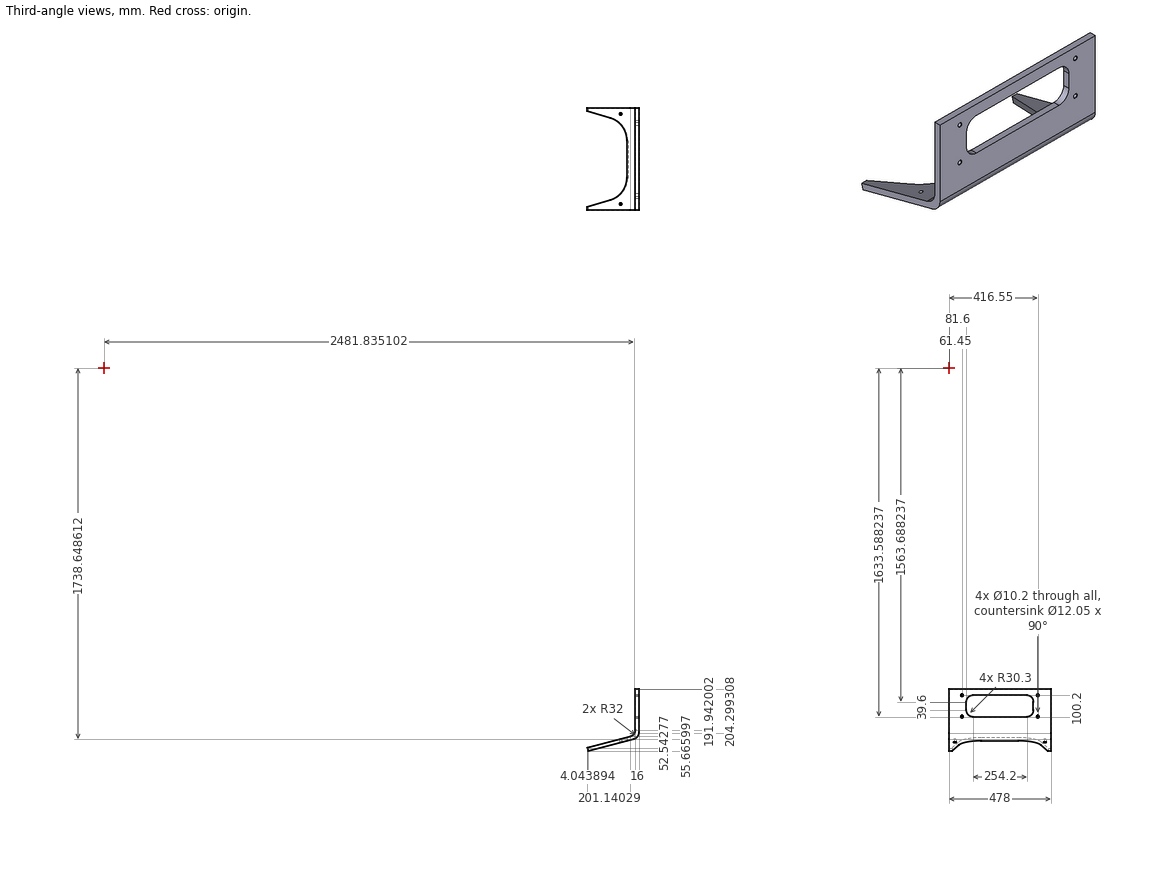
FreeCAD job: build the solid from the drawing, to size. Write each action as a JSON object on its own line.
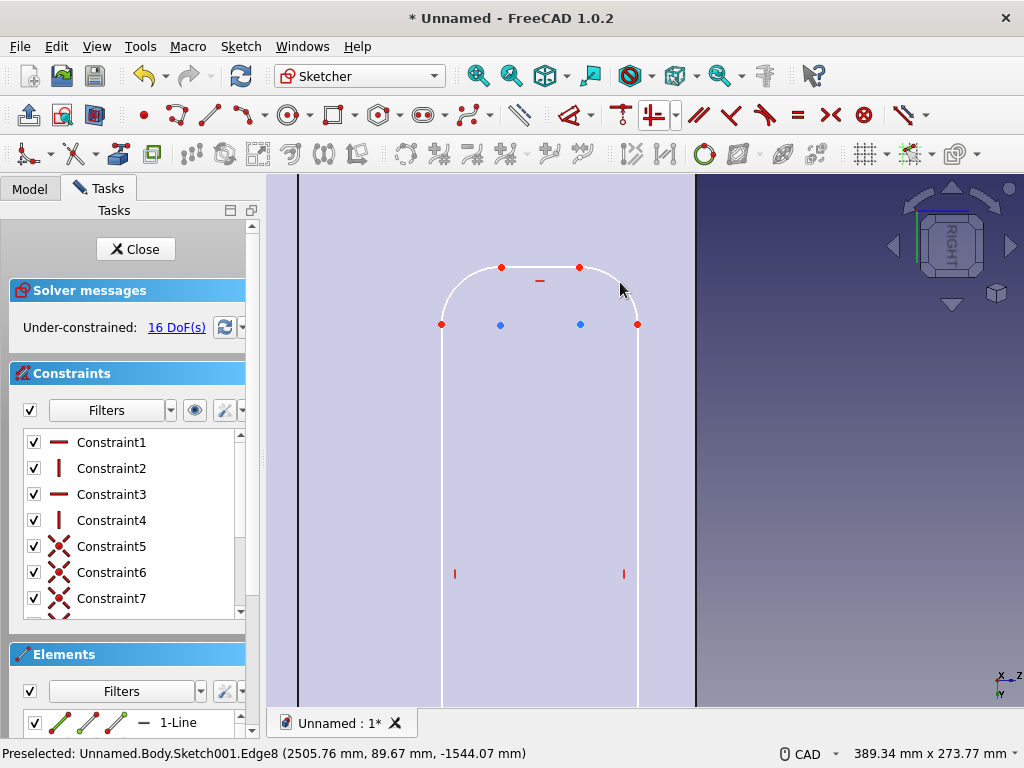
{"action": "left_click", "coordinate": [556, 267]}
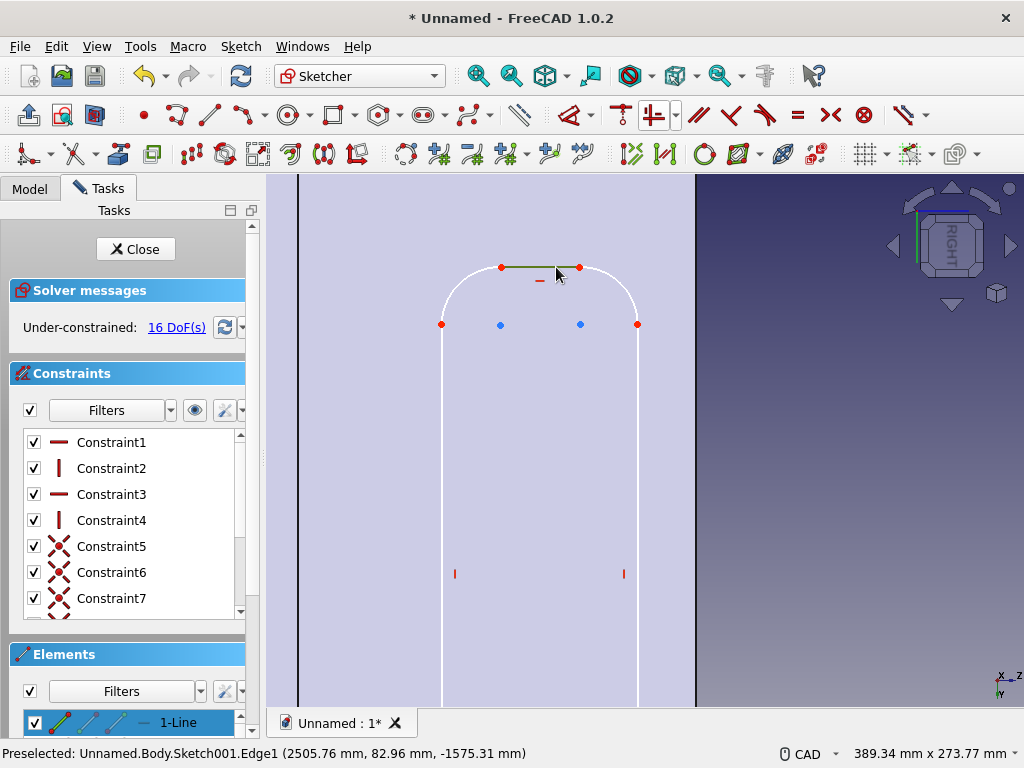
{"action": "left_click", "coordinate": [475, 273]}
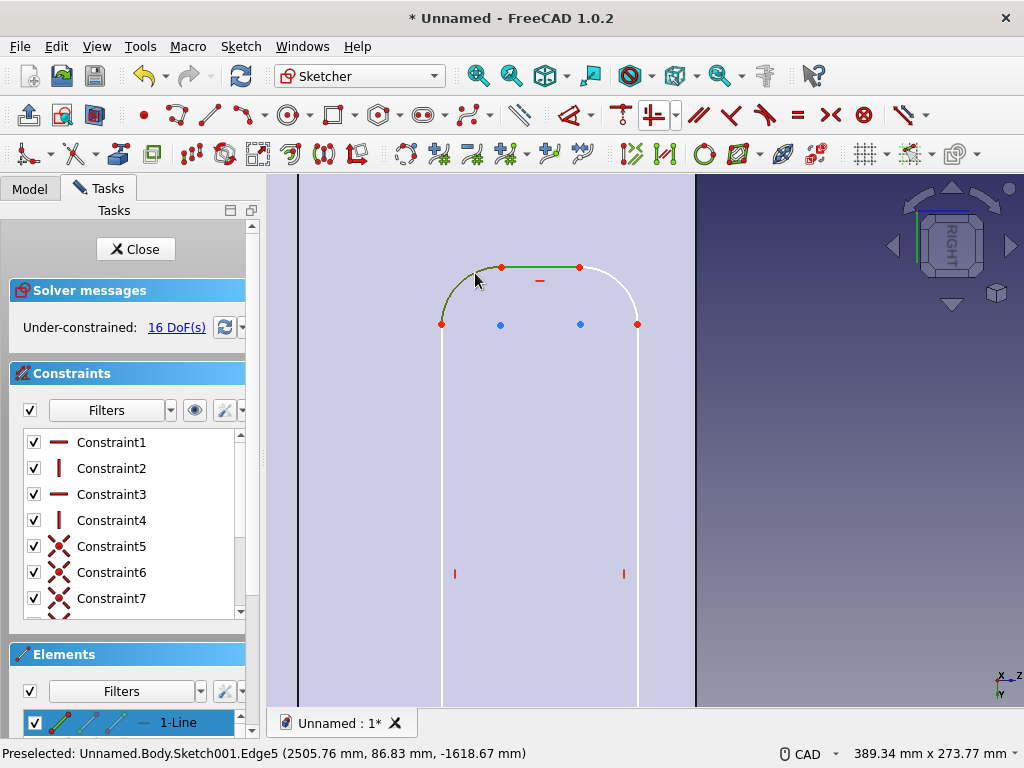
{"action": "left_click", "coordinate": [765, 116]}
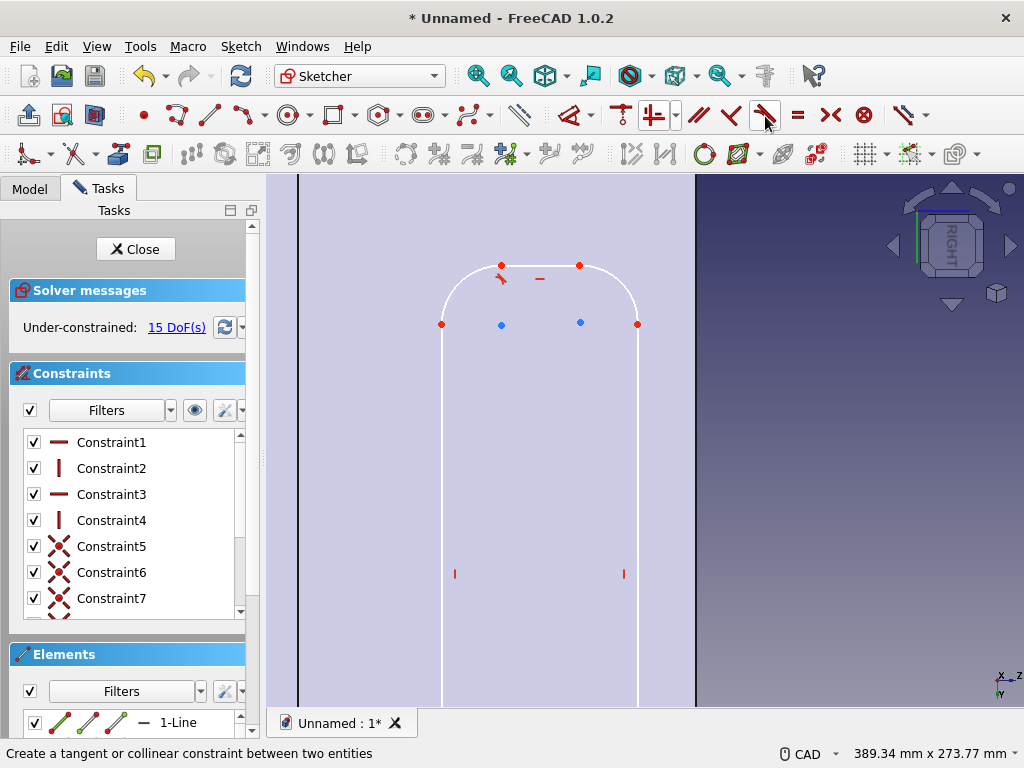
{"action": "left_click", "coordinate": [556, 266]}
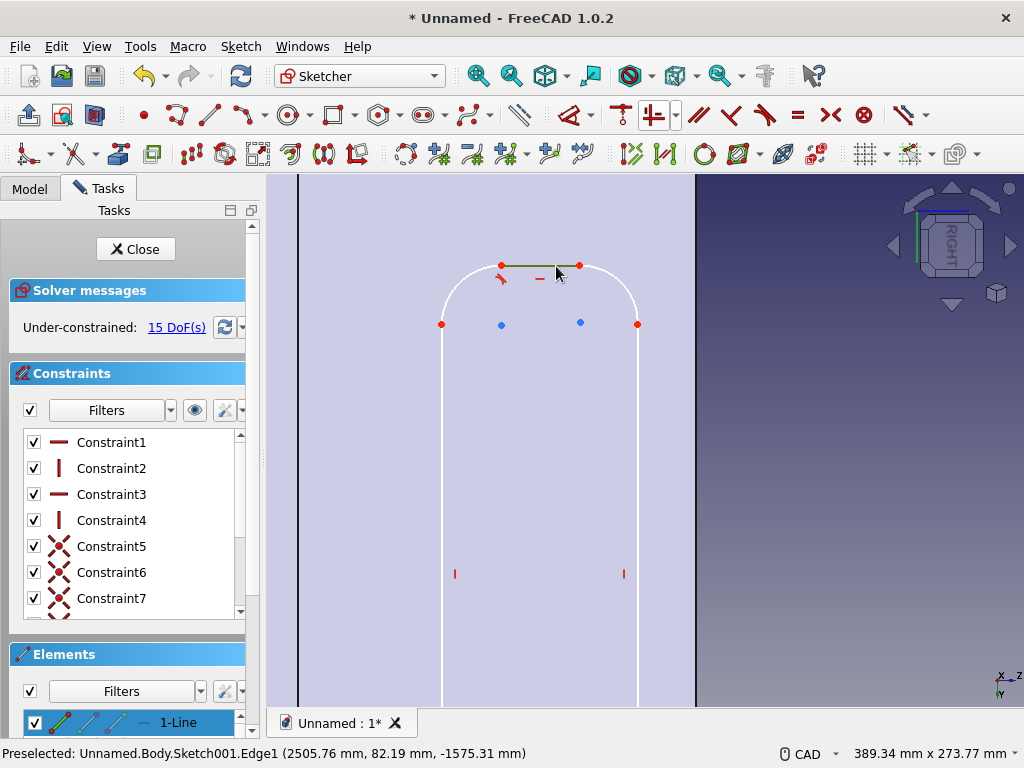
{"action": "left_click", "coordinate": [632, 298]}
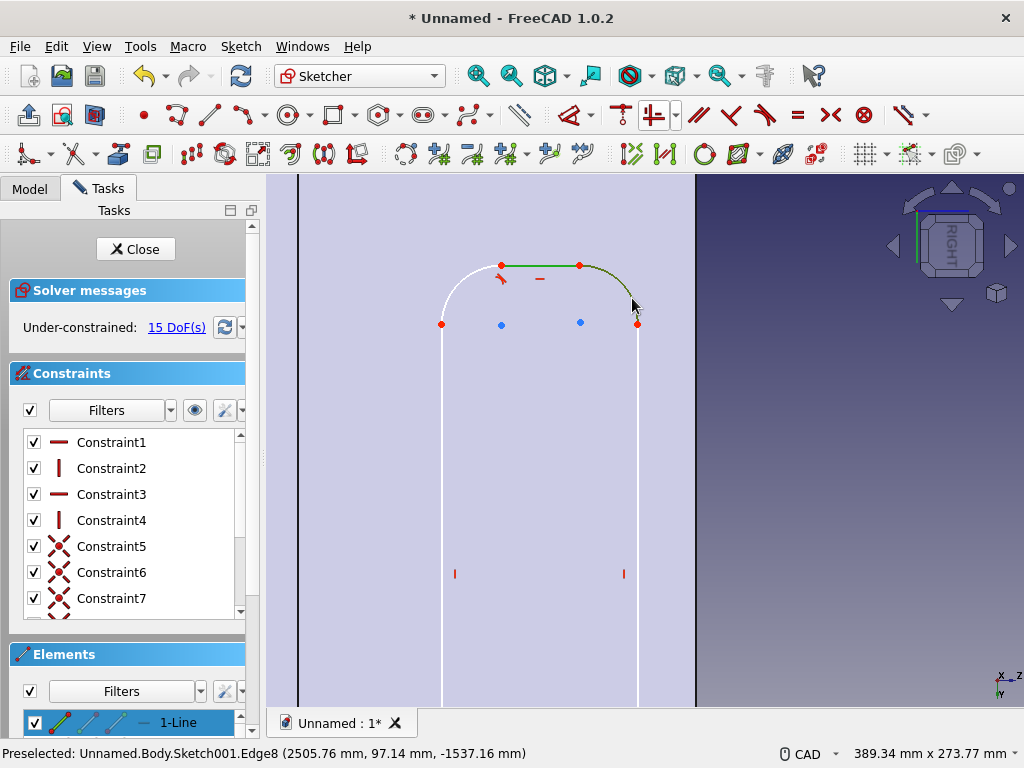
{"action": "left_click", "coordinate": [765, 116]}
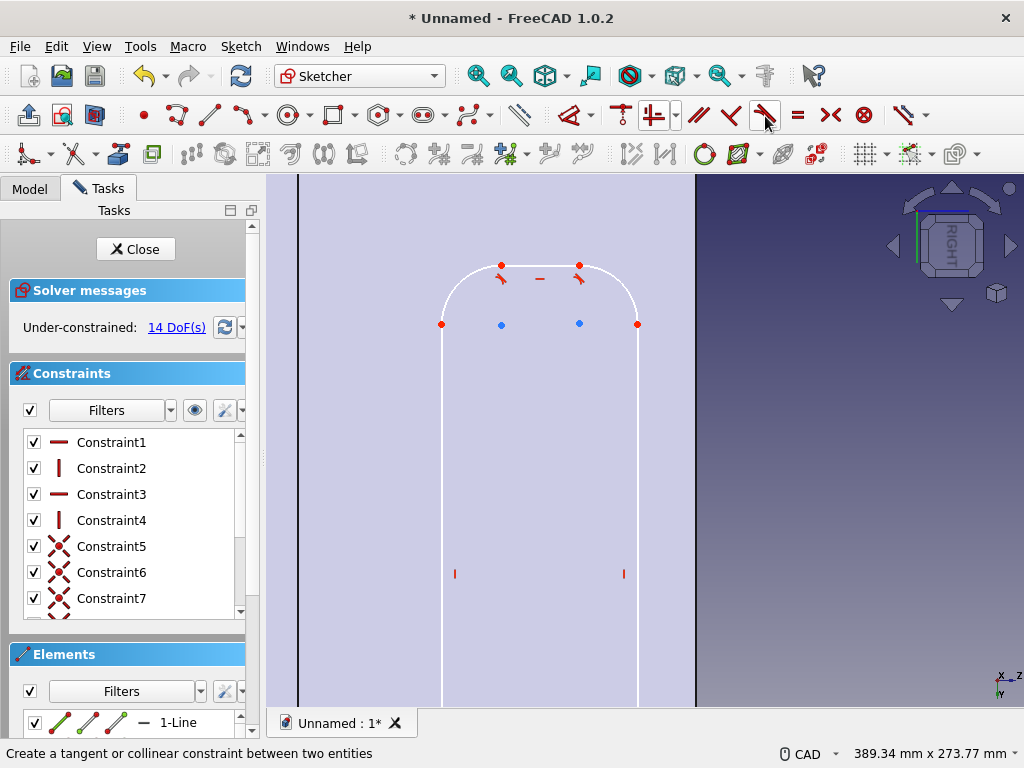
{"action": "left_click", "coordinate": [442, 474]}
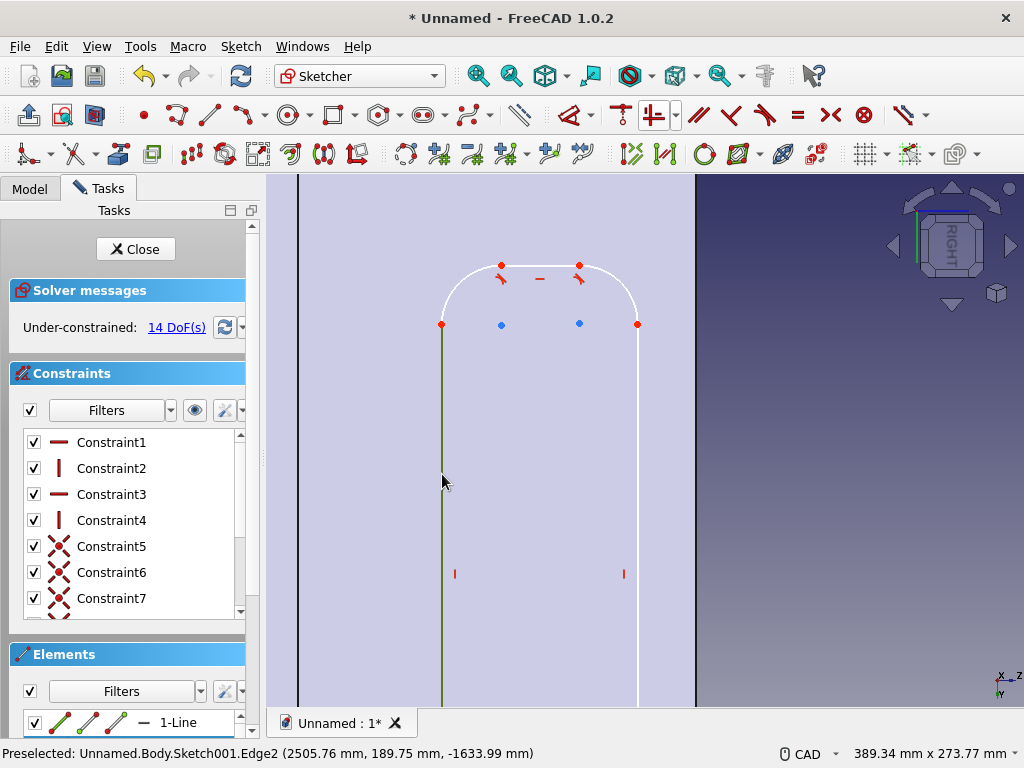
{"action": "left_click", "coordinate": [475, 272]}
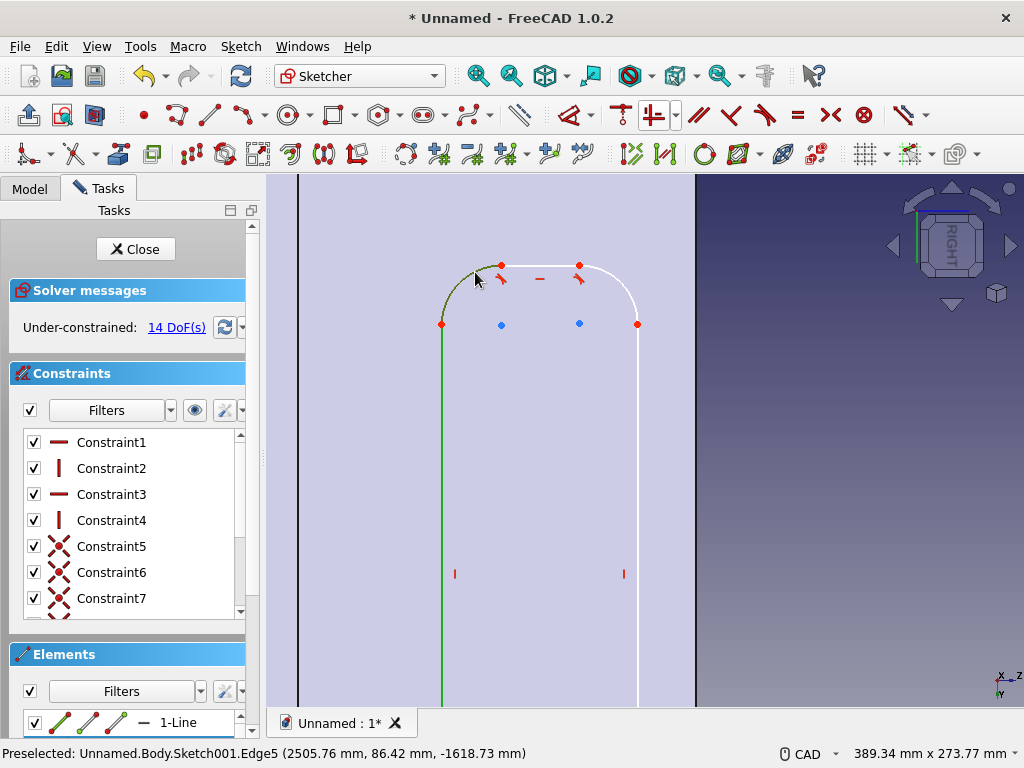
{"action": "left_click", "coordinate": [765, 116]}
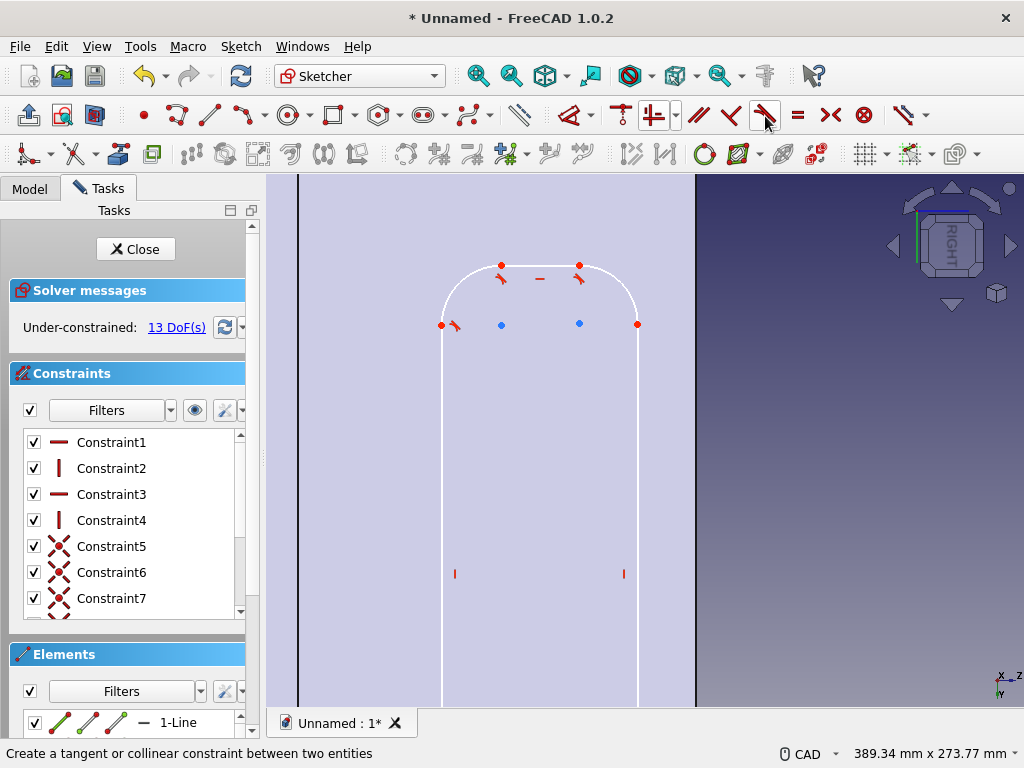
{"action": "left_click", "coordinate": [442, 474]}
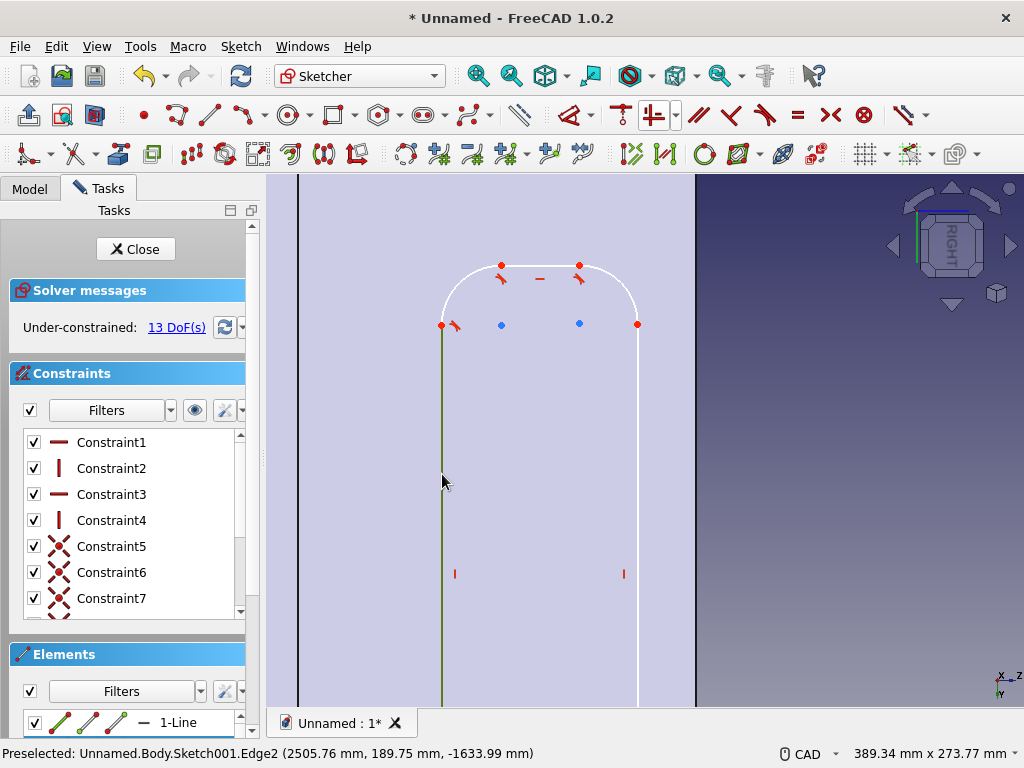
{"action": "scroll", "coordinate": [621, 282], "scroll_direction": "down", "scroll_amount": 3}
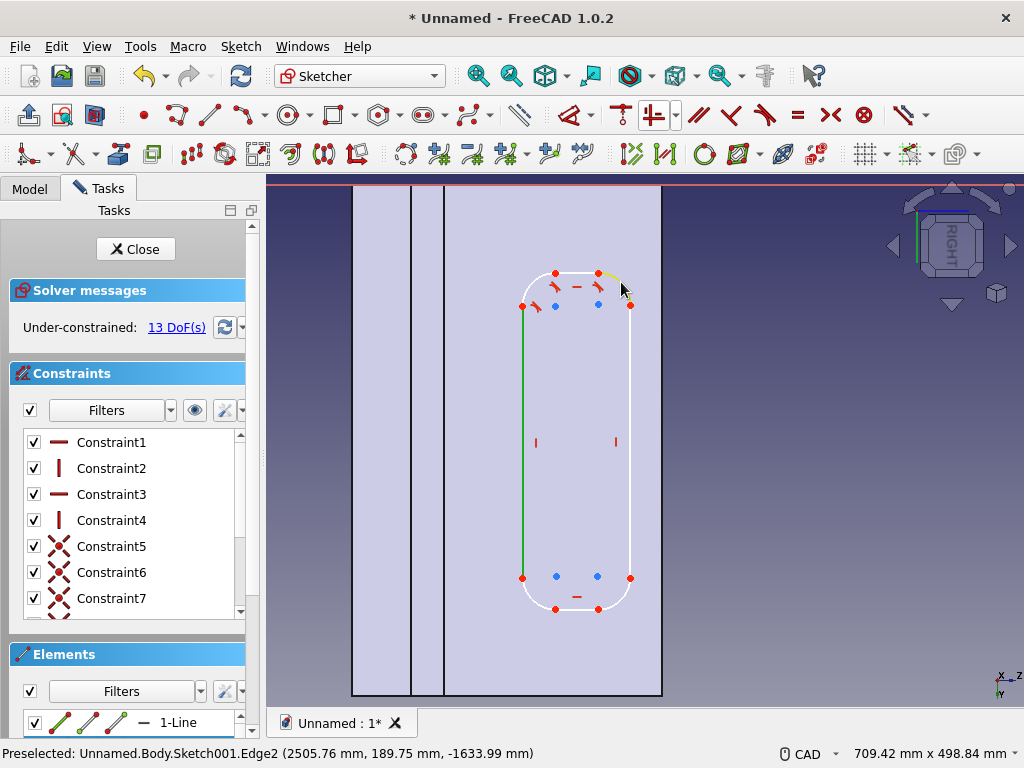
{"action": "left_click", "coordinate": [527, 592]}